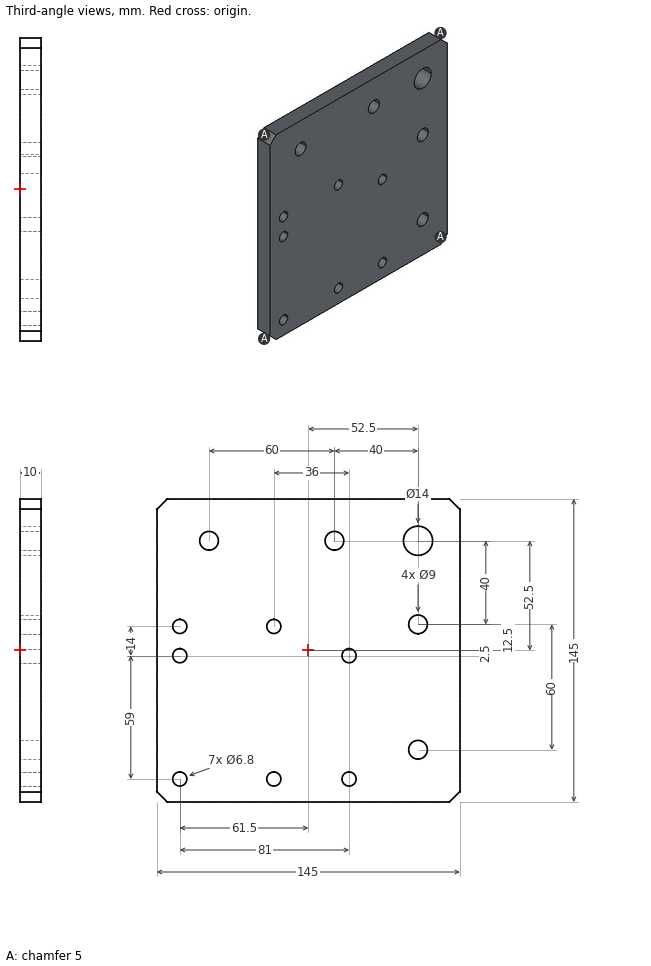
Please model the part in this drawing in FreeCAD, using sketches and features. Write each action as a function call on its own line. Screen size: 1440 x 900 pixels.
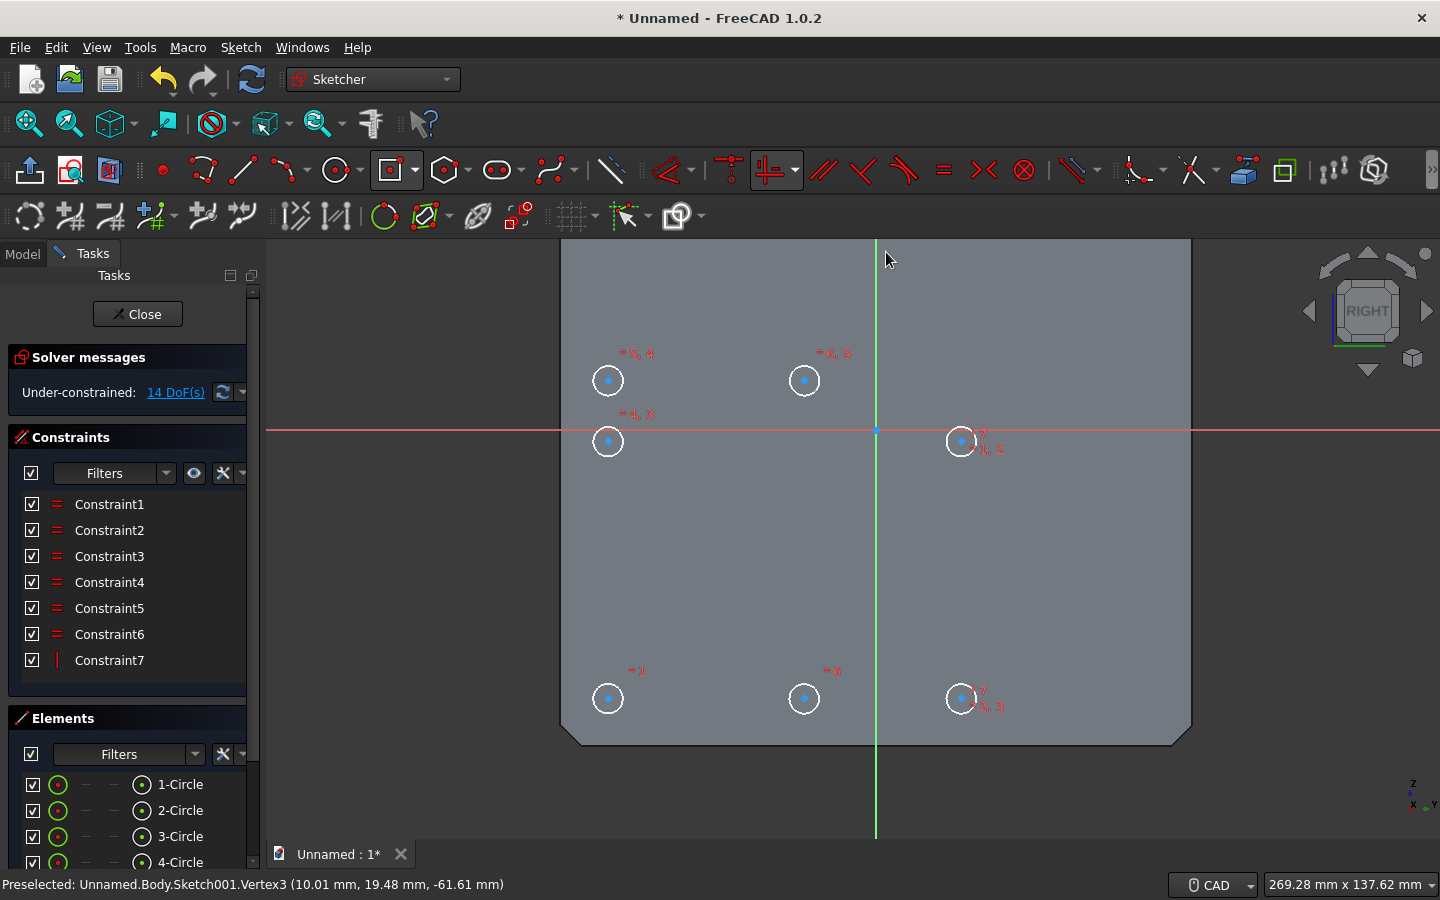
click(608, 699)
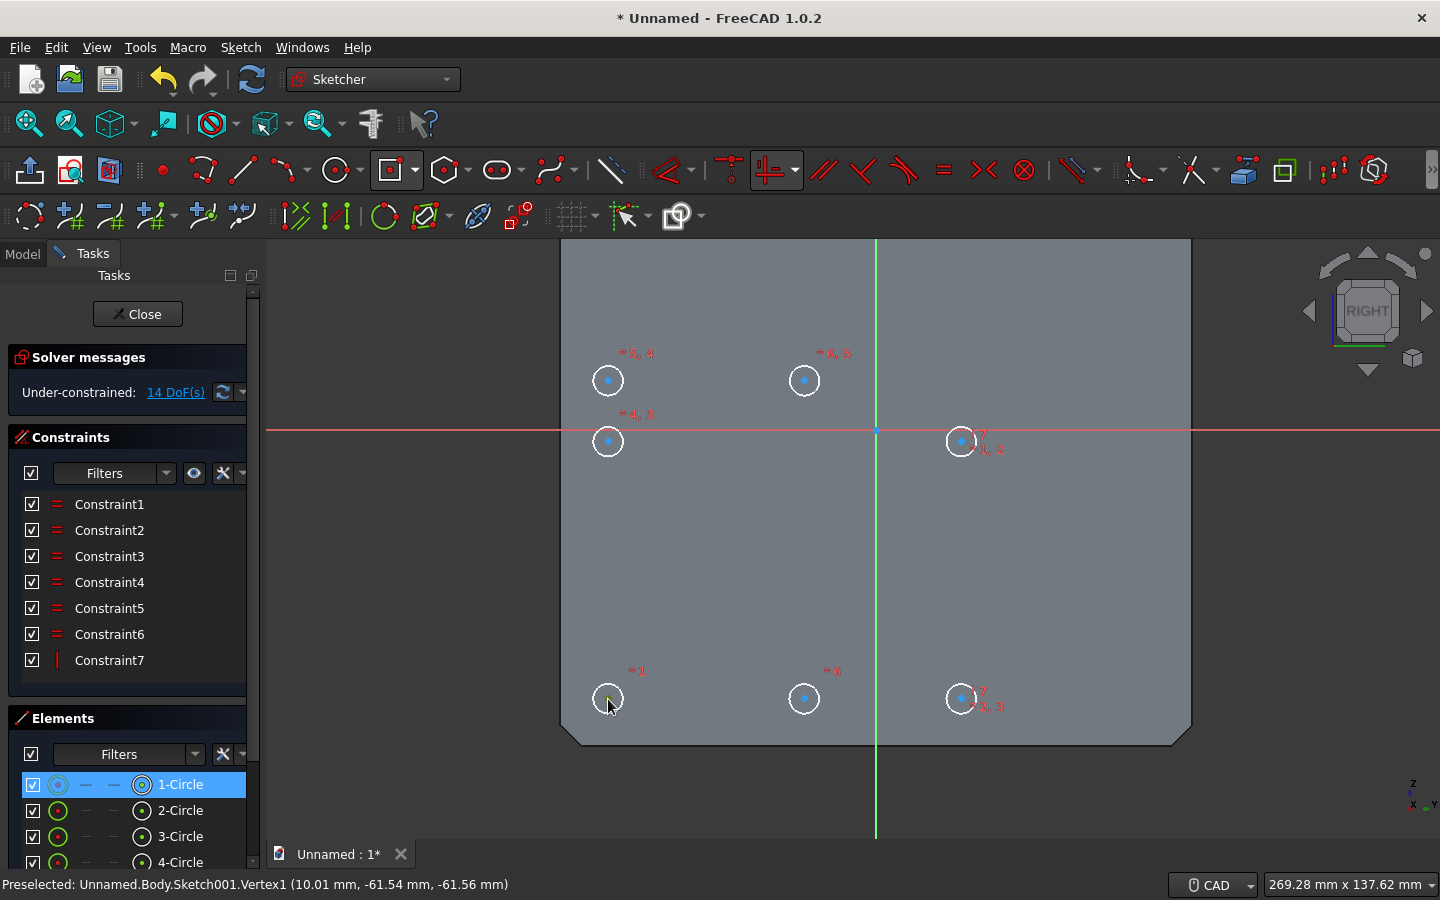
click(961, 699)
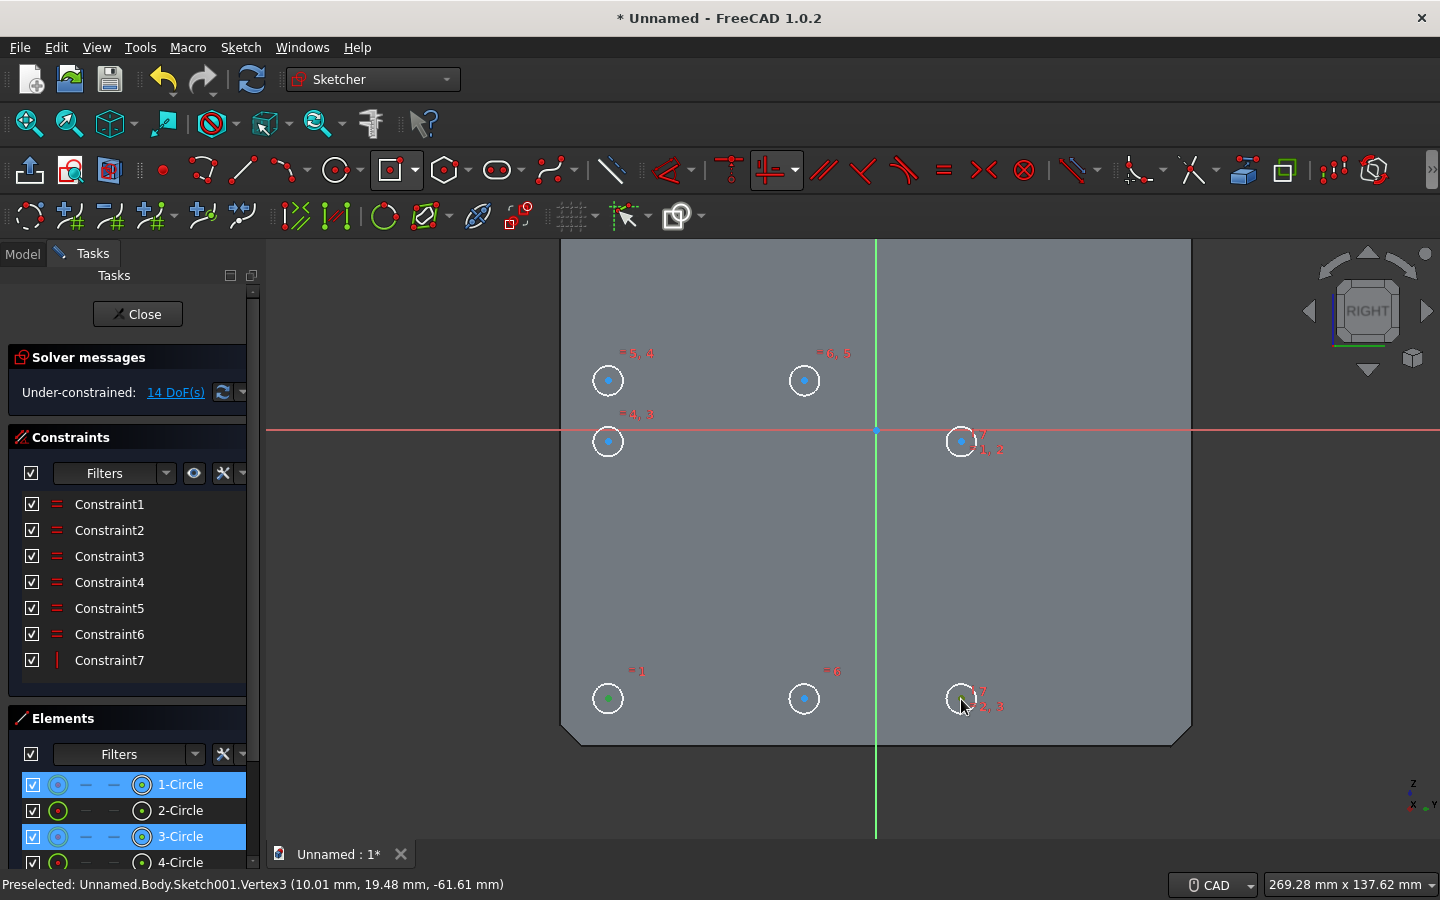
key(h)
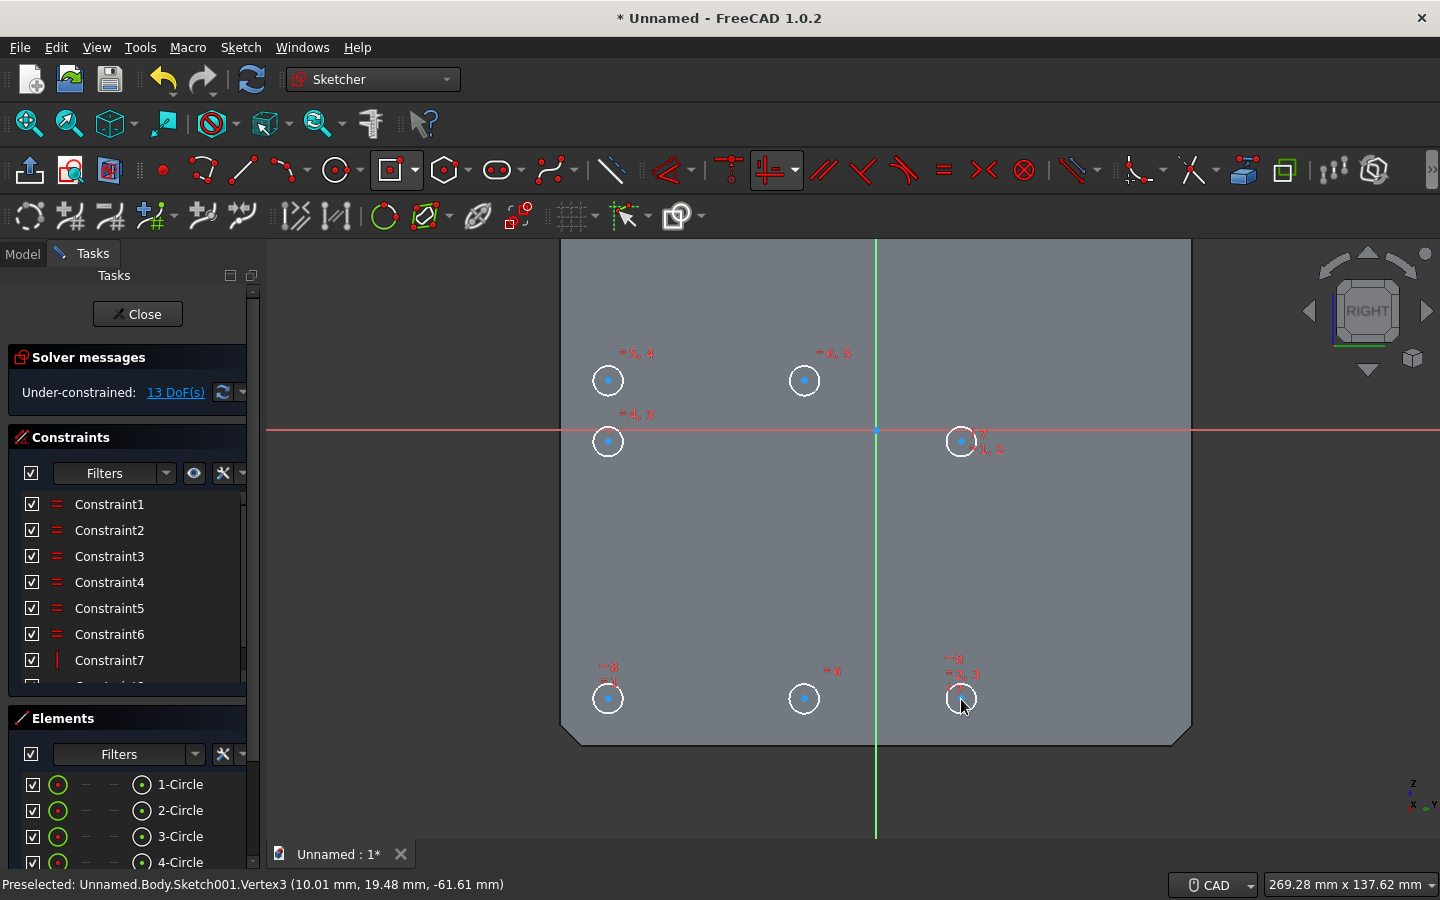
click(608, 699)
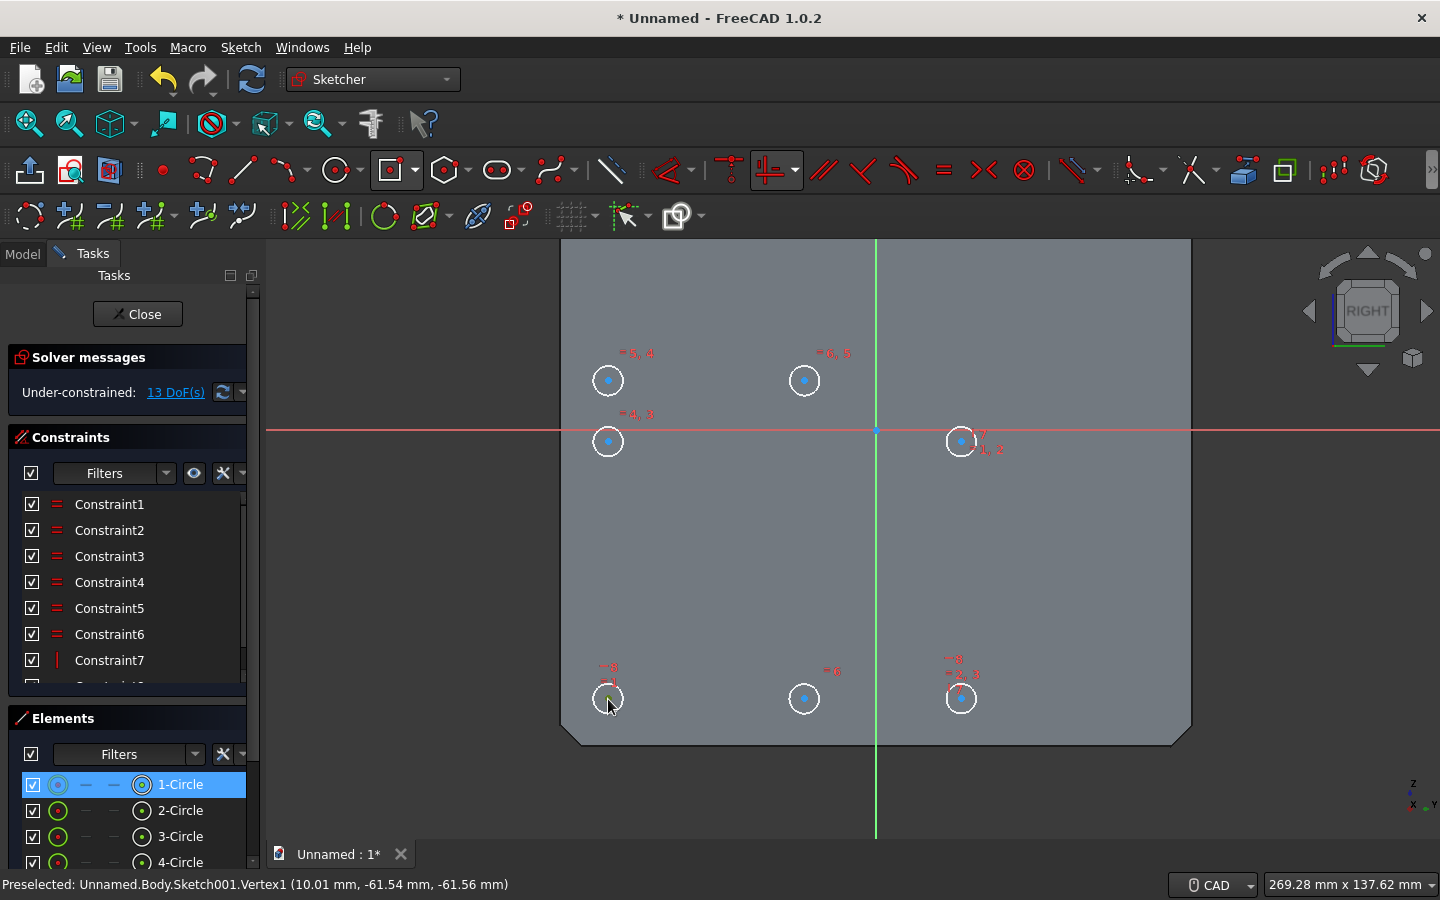
click(608, 442)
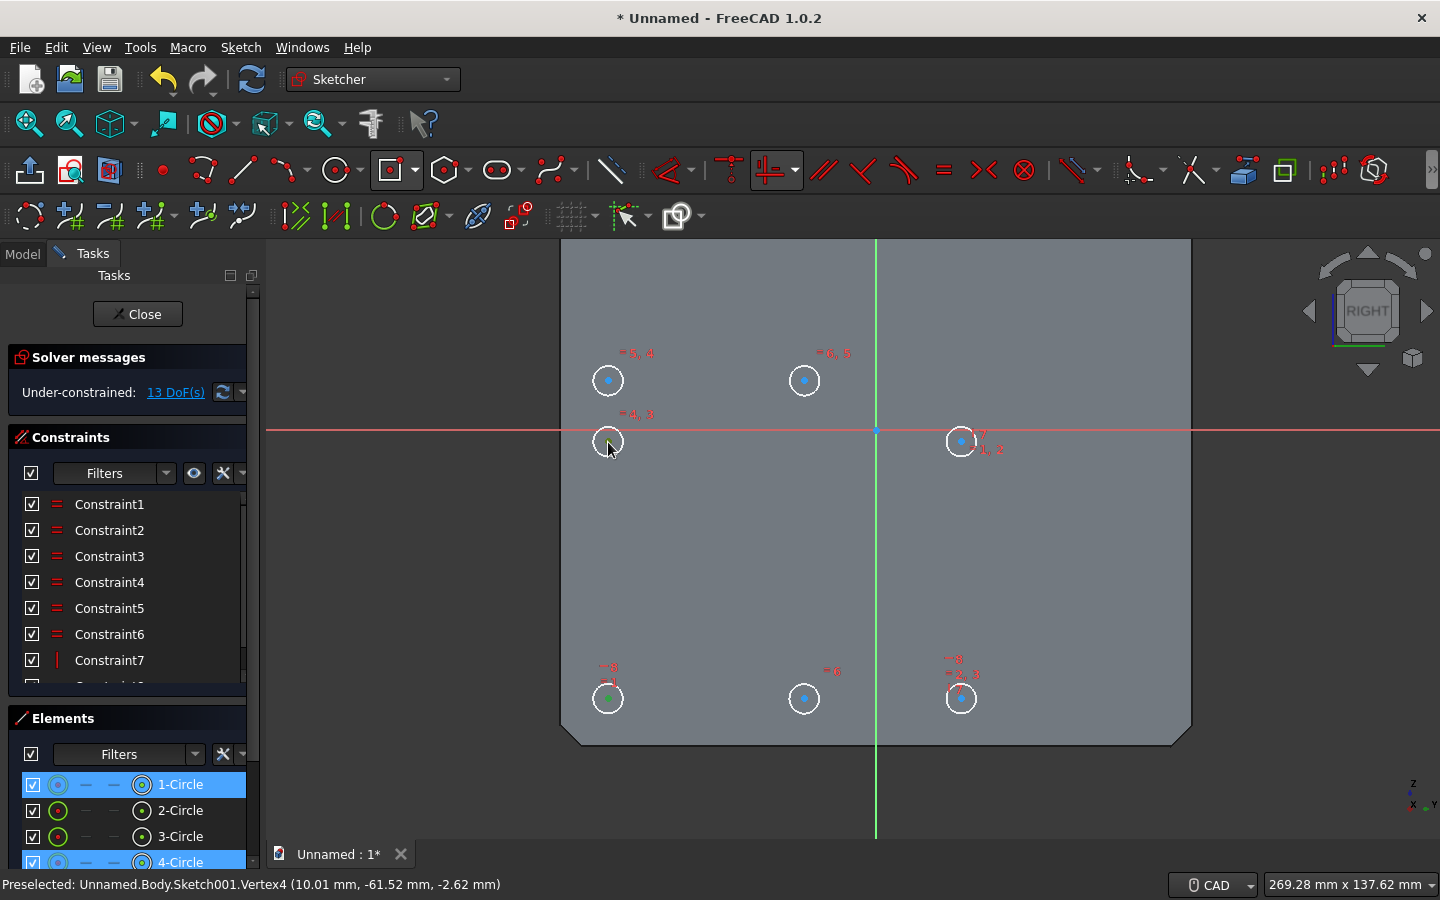
key(v)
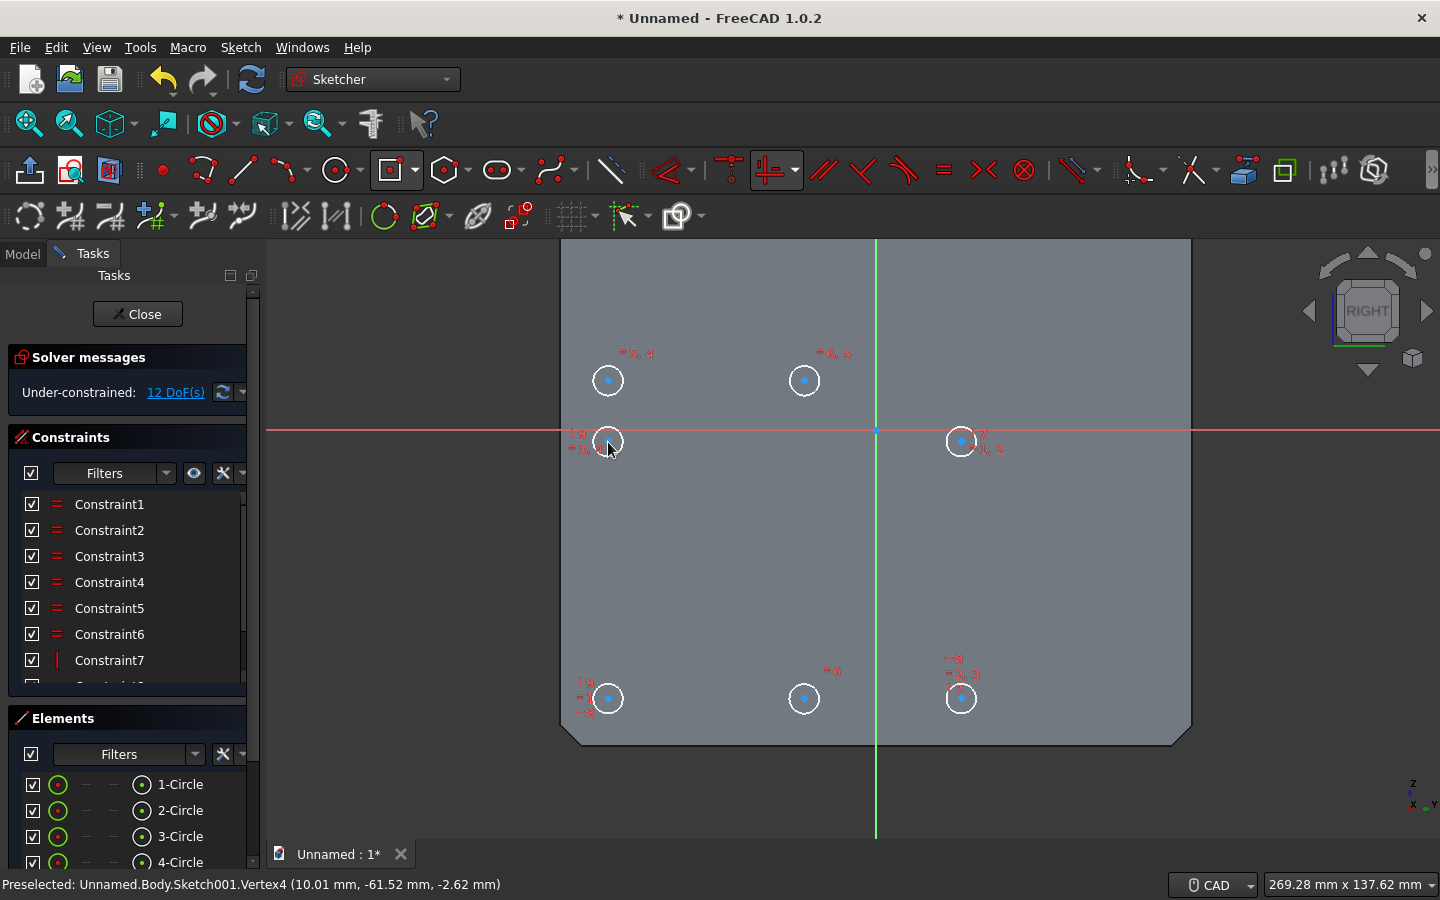
click(961, 442)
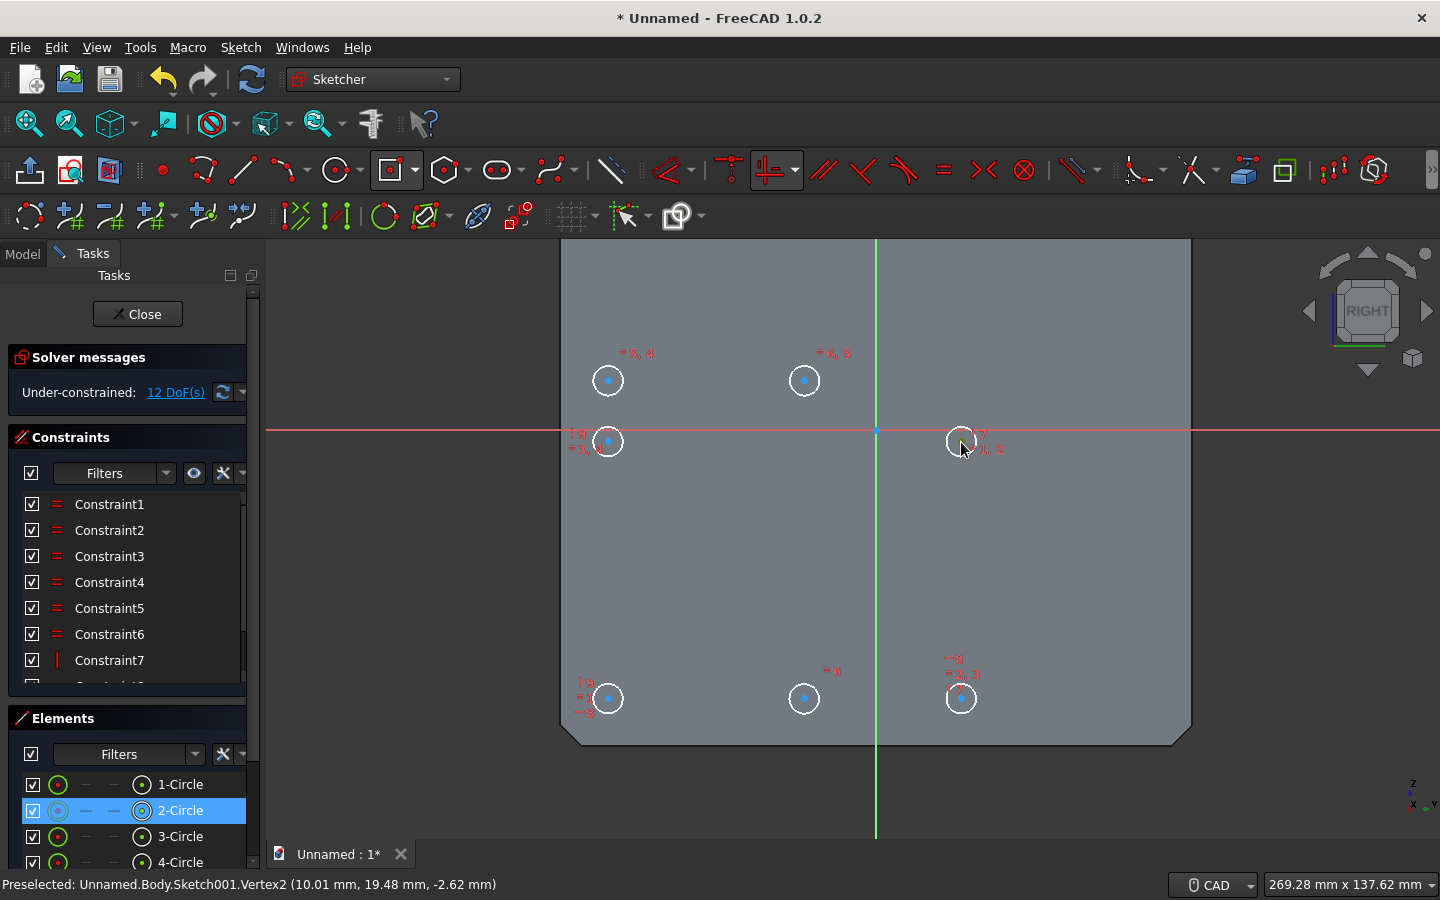
click(608, 442)